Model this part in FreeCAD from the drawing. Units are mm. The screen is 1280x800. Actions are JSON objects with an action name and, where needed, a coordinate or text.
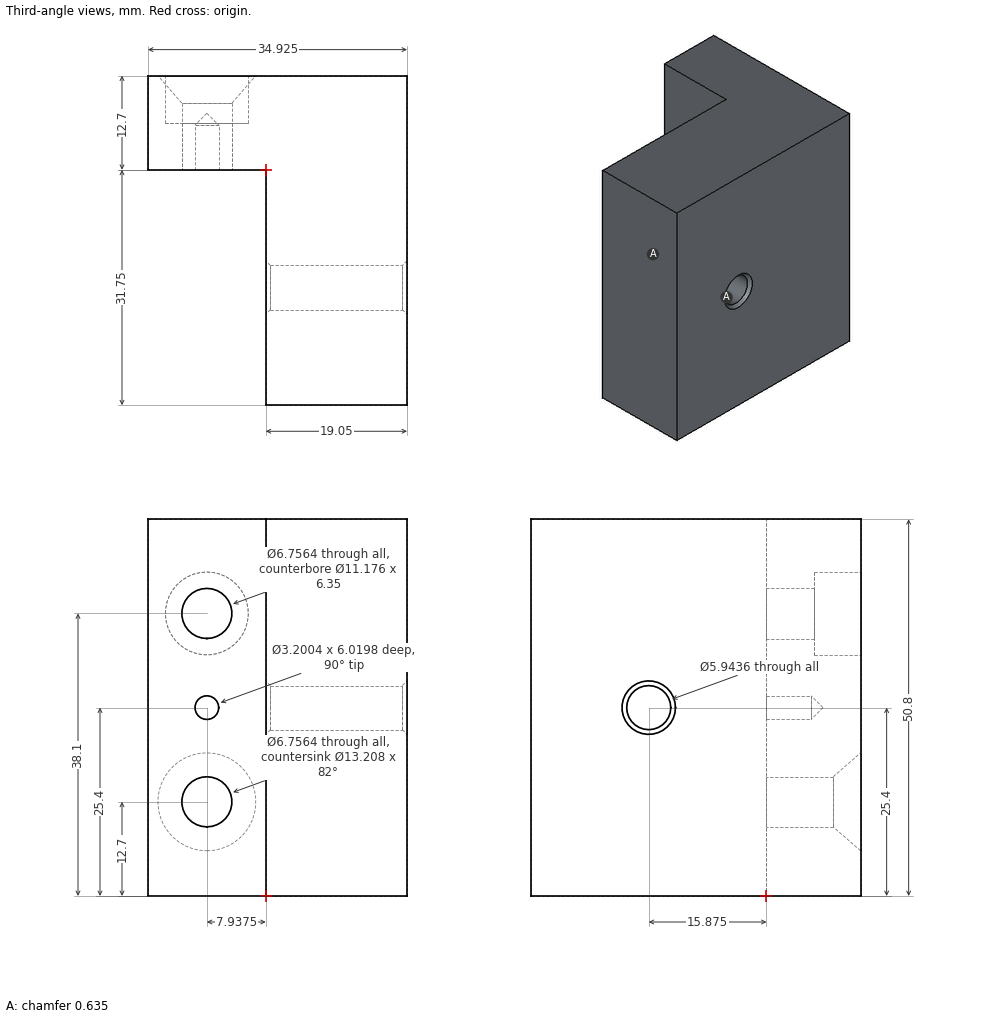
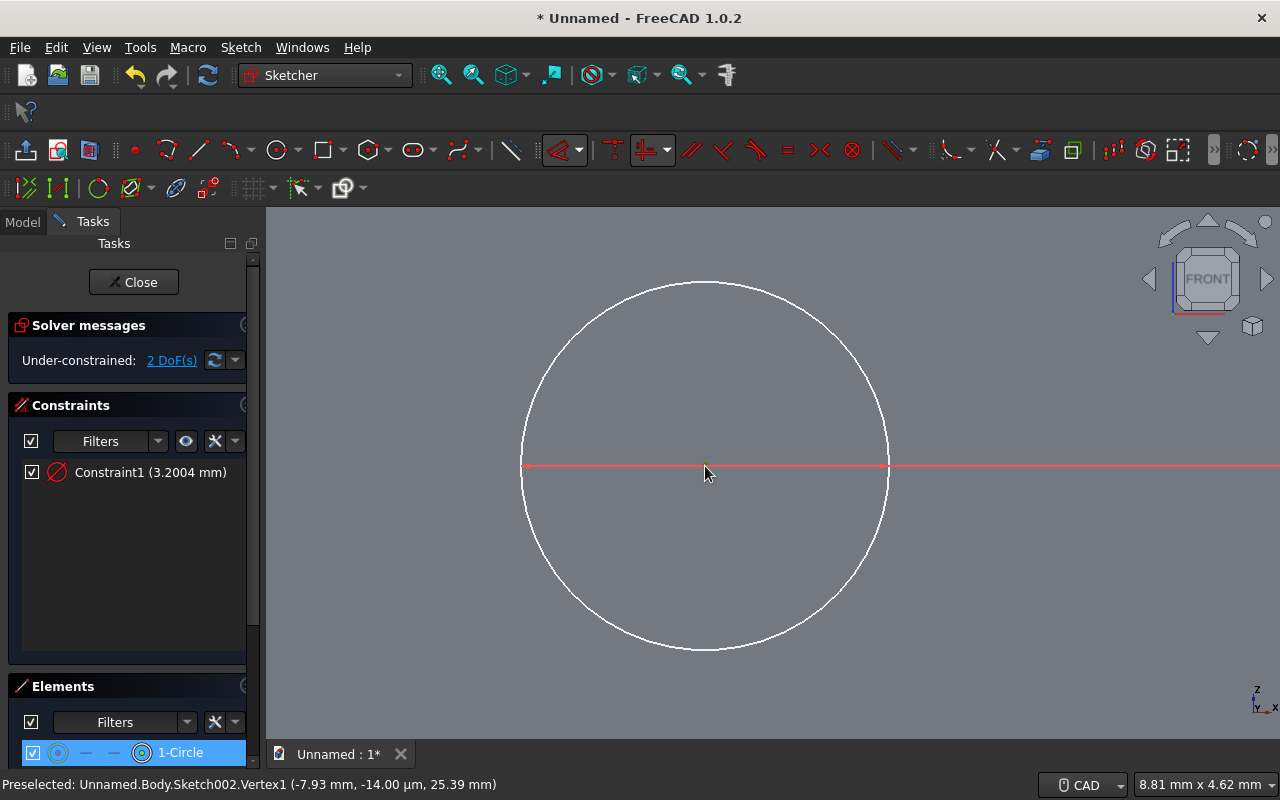
{"action": "key", "text": "i"}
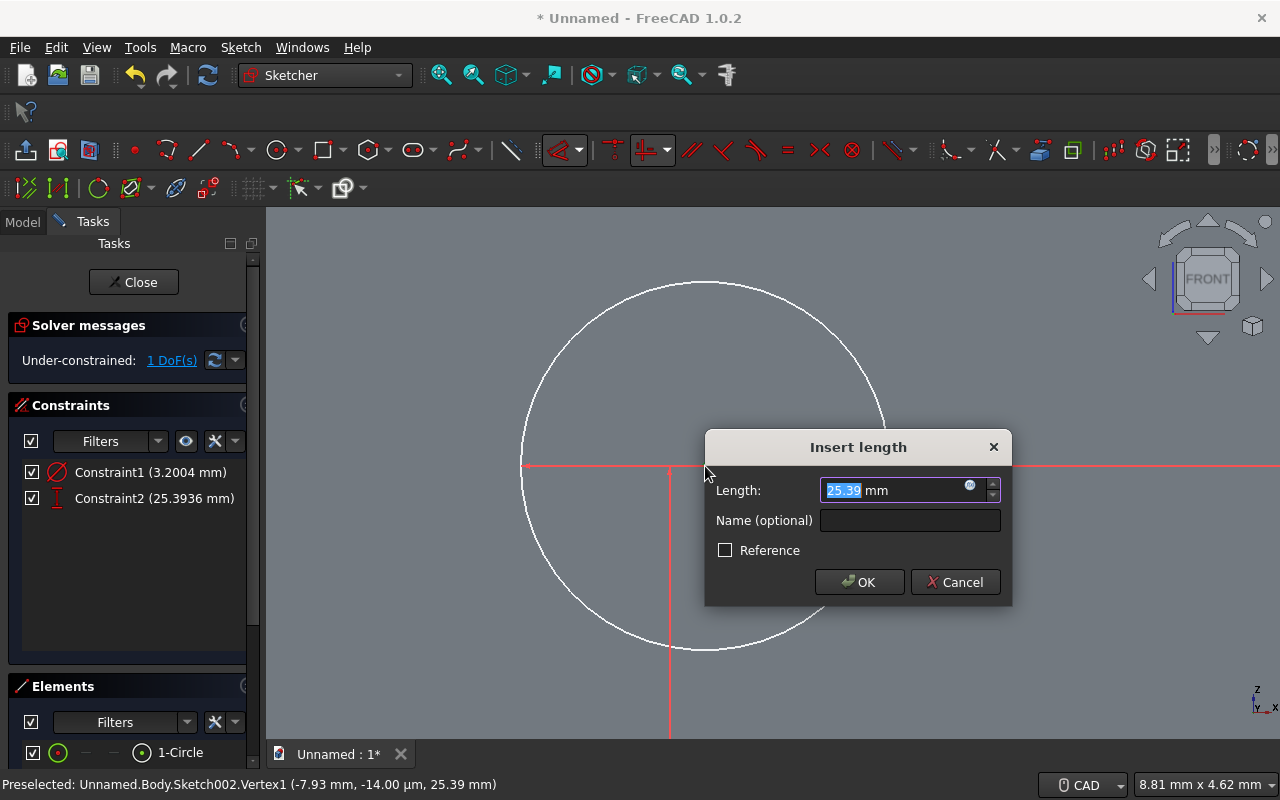
{"action": "type", "text": "25.4"}
{"action": "key", "text": "Return"}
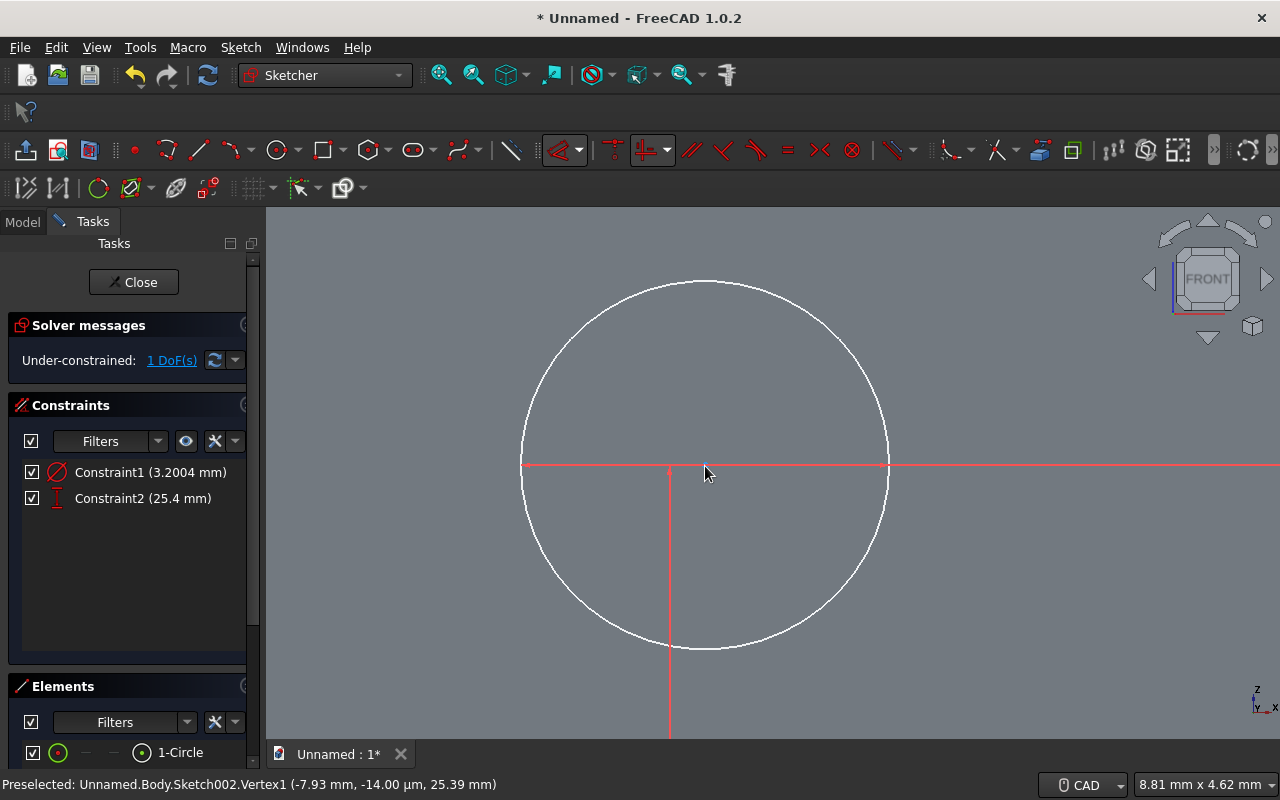
{"action": "left_click", "coordinate": [705, 465]}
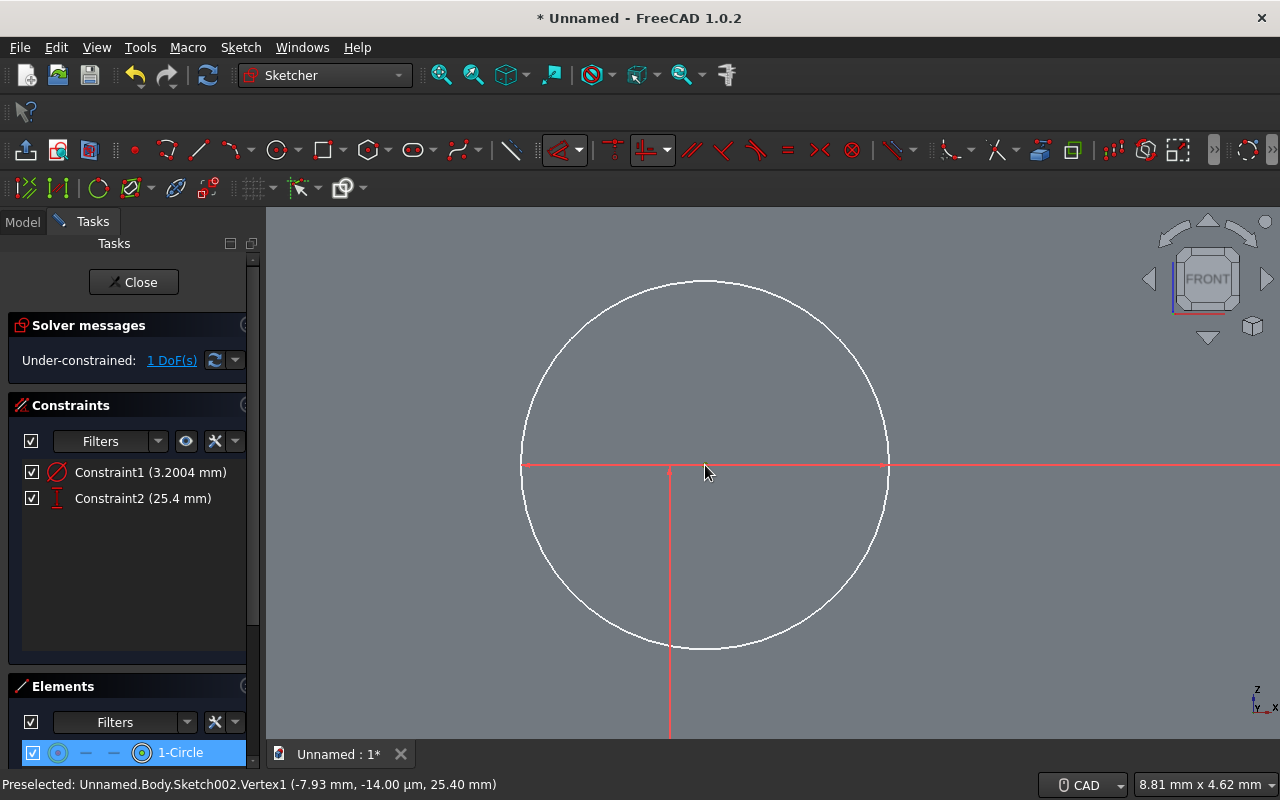
{"action": "left_click", "coordinate": [582, 150]}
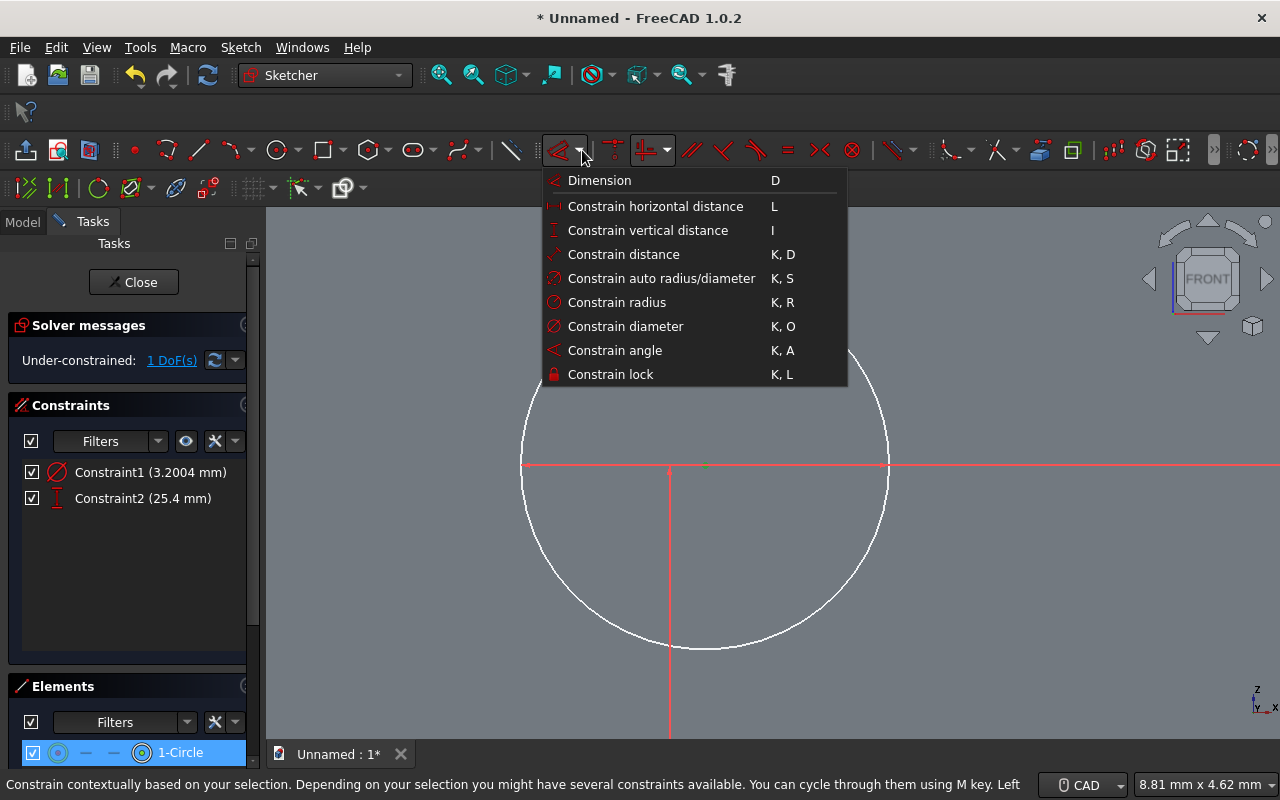
{"action": "left_click", "coordinate": [695, 206]}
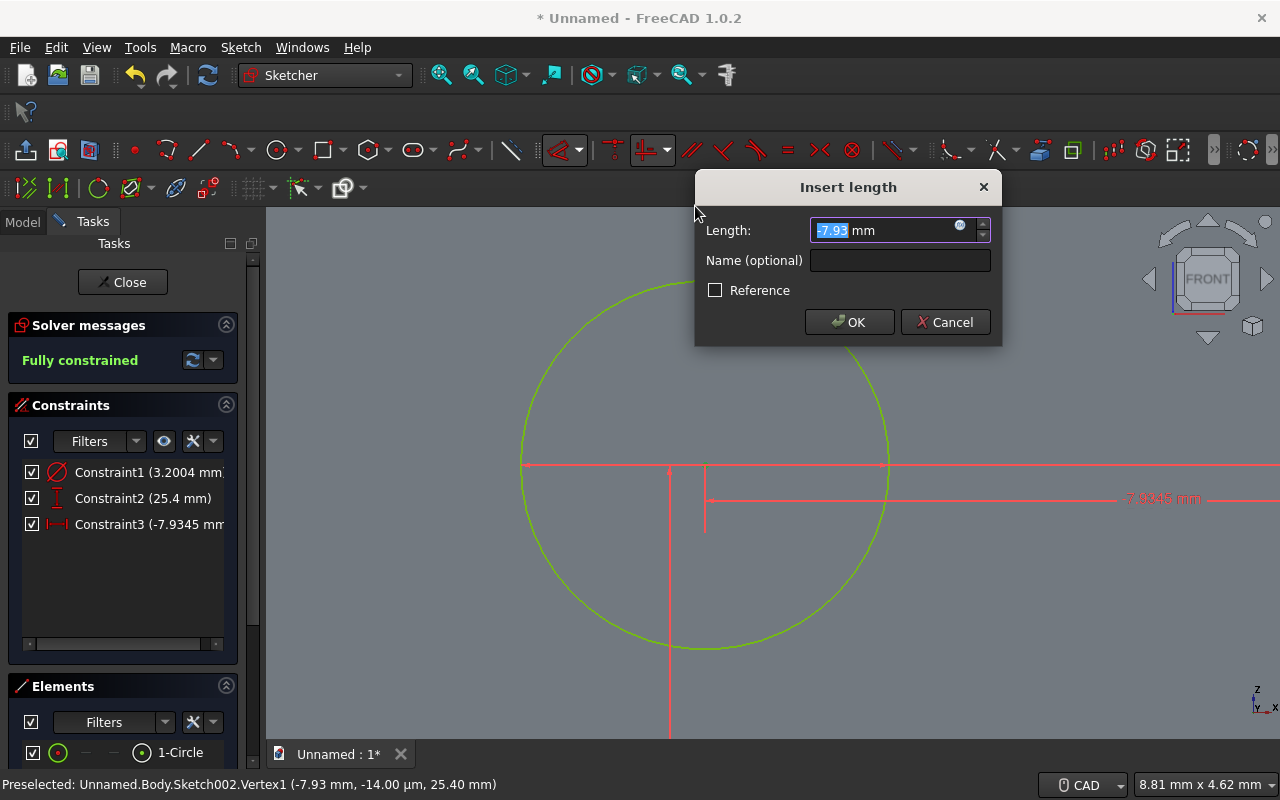
{"action": "type", "text": "-7.9375"}
{"action": "key", "text": "Return"}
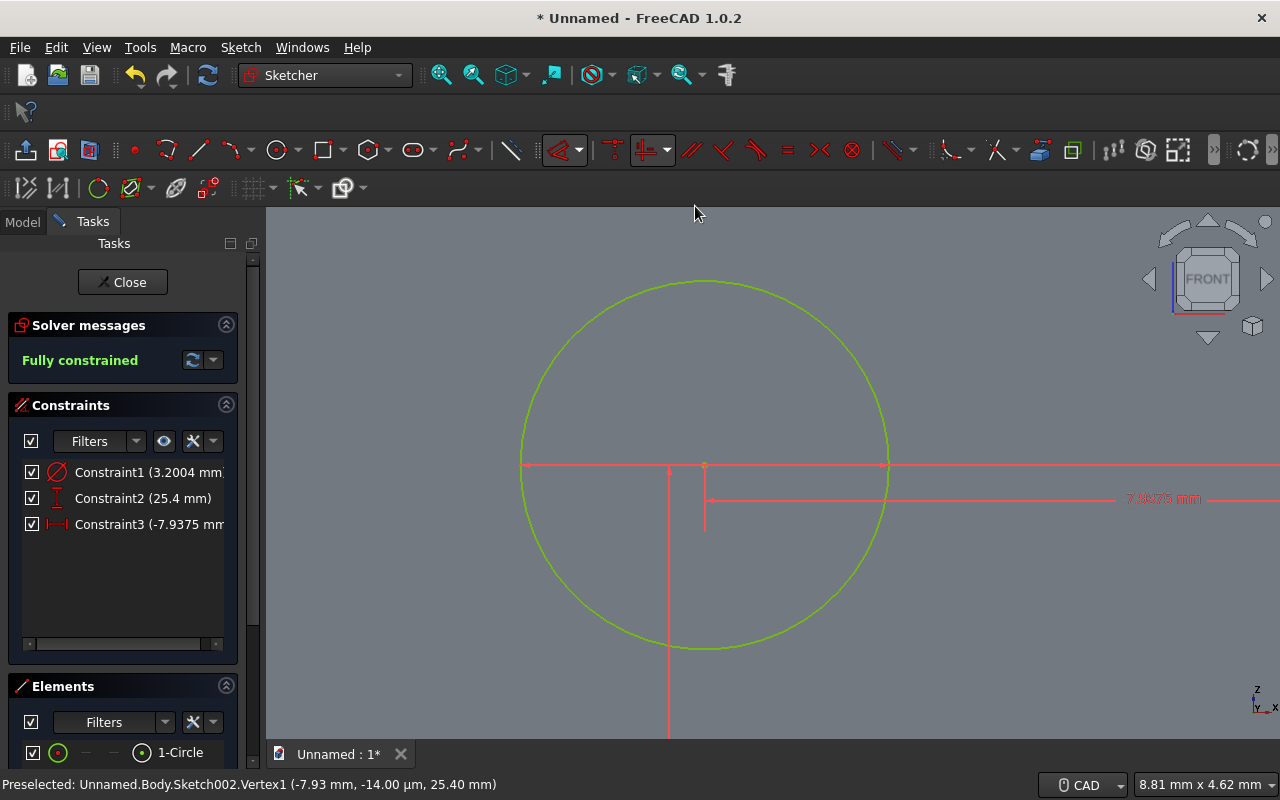
{"action": "left_click", "coordinate": [123, 282]}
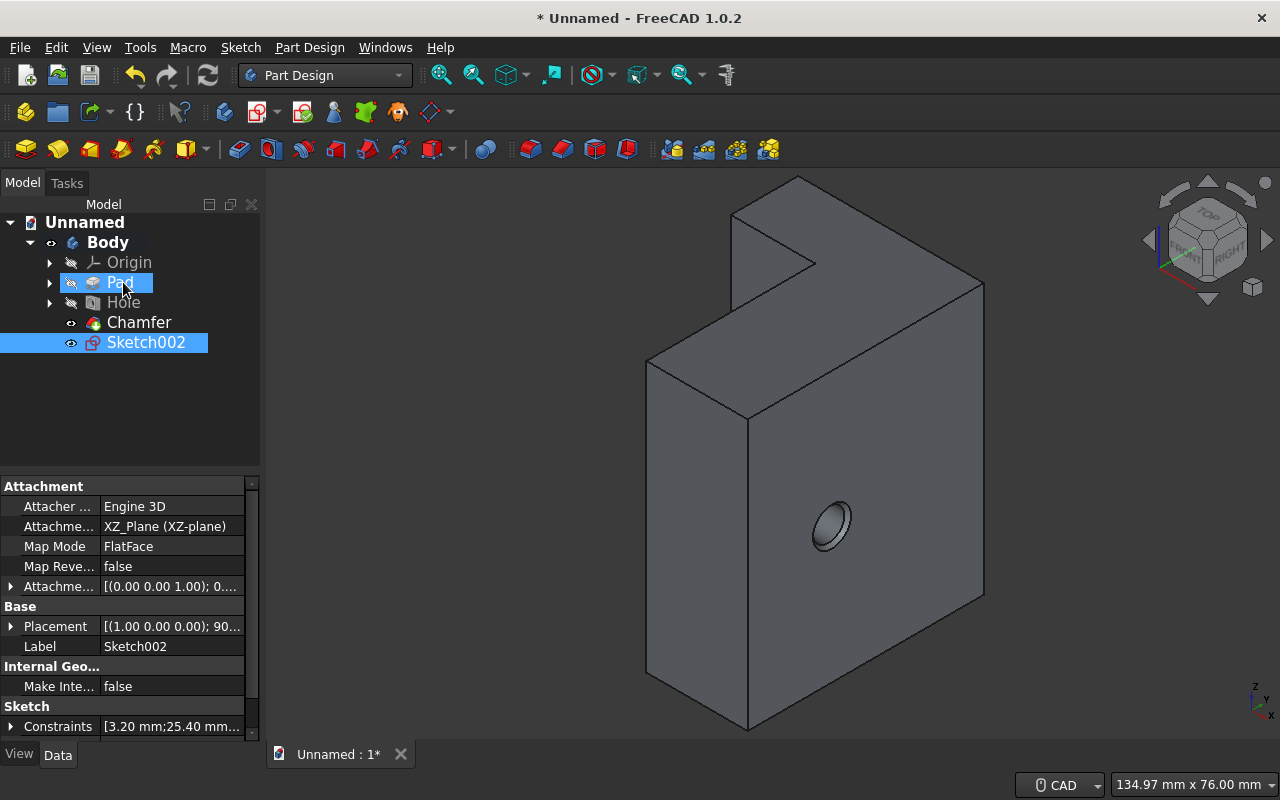
{"action": "left_click", "coordinate": [272, 150]}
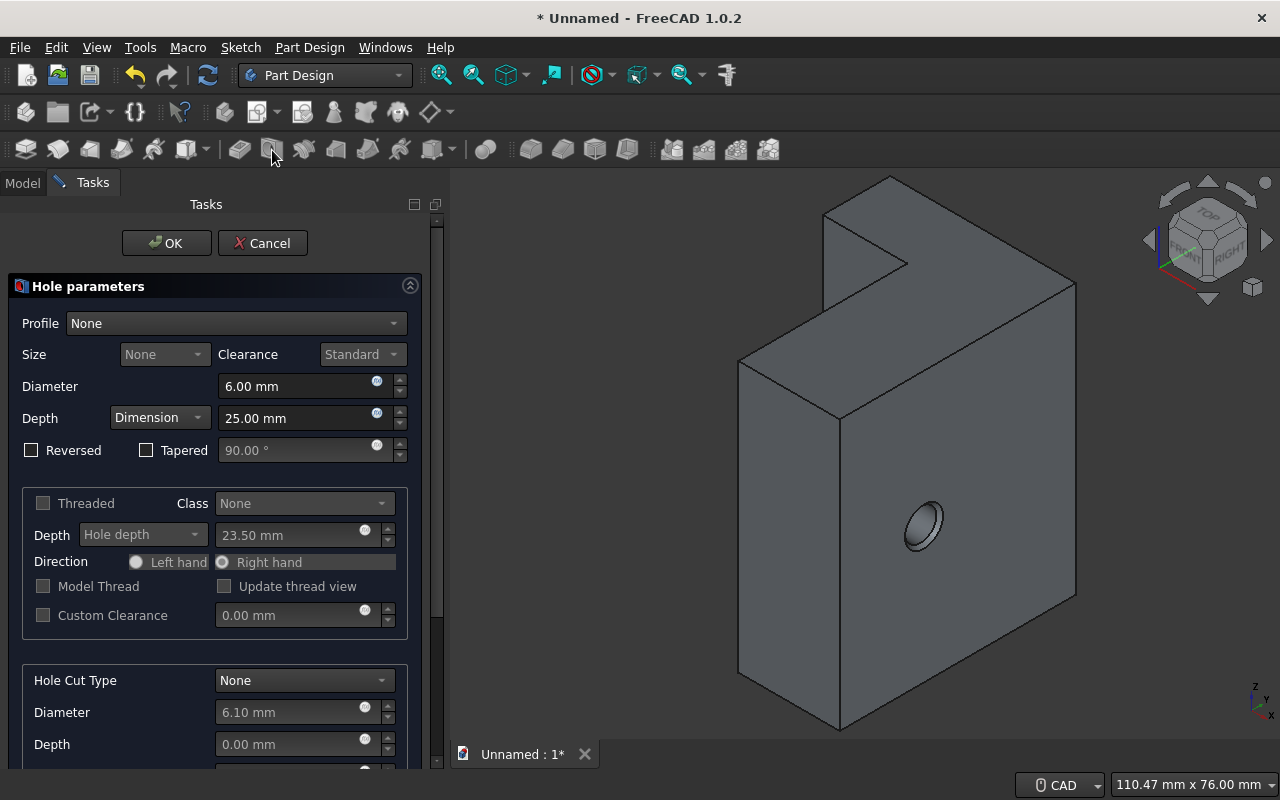
{"action": "triple_click", "coordinate": [305, 386]}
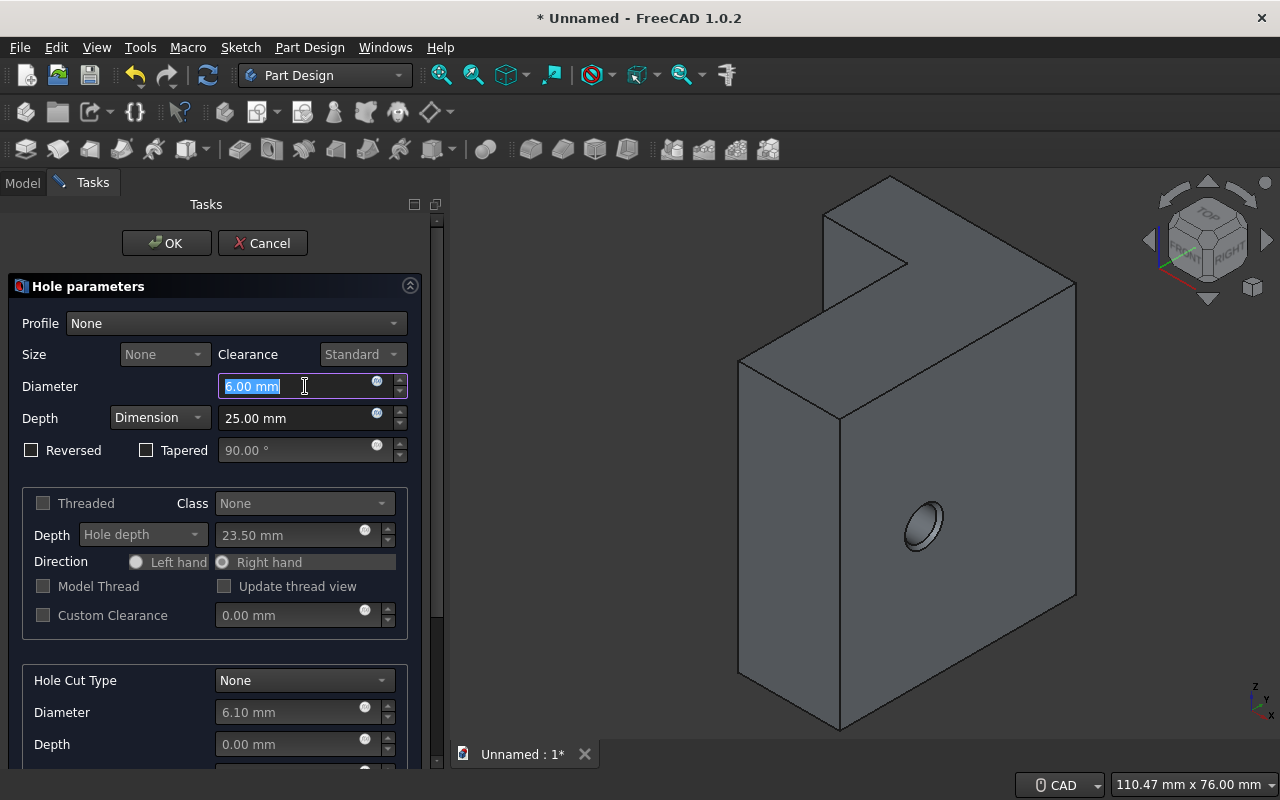
{"action": "type", "text": "3.2004"}
{"action": "key", "text": "Tab"}